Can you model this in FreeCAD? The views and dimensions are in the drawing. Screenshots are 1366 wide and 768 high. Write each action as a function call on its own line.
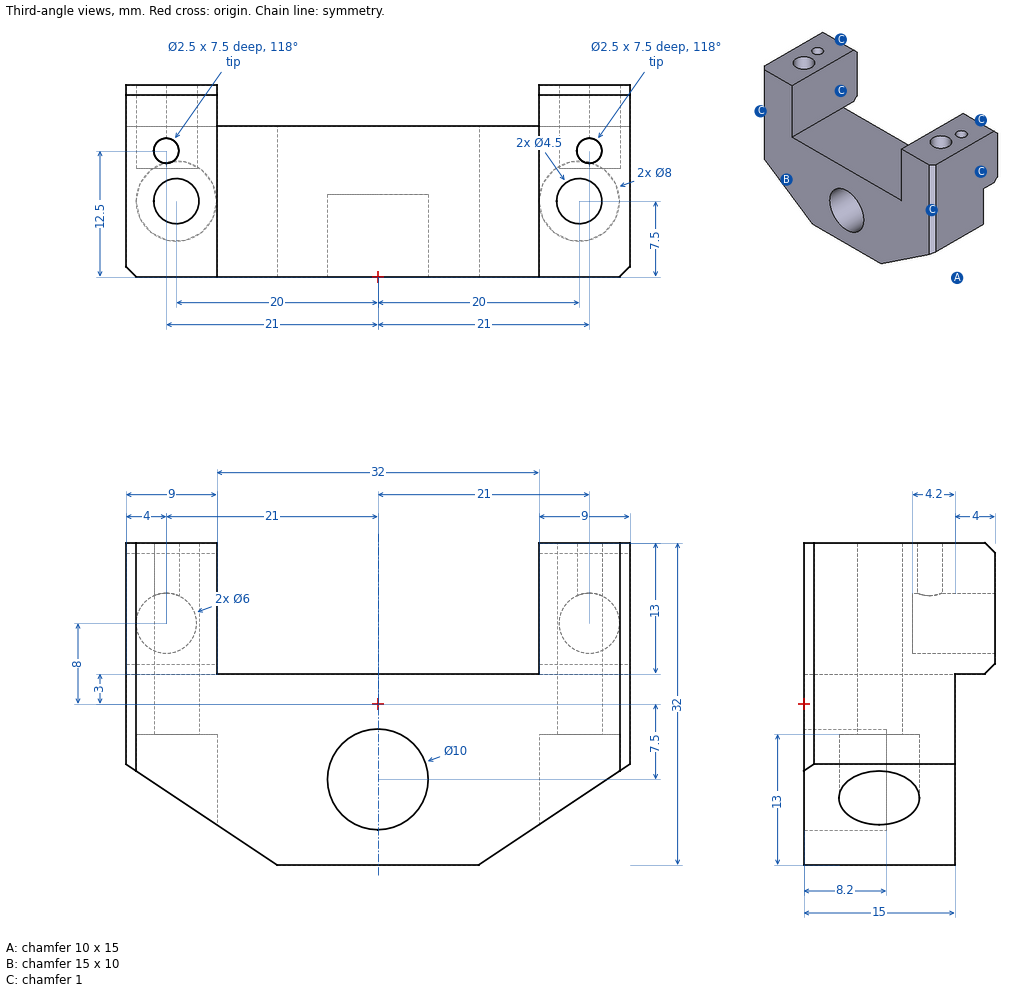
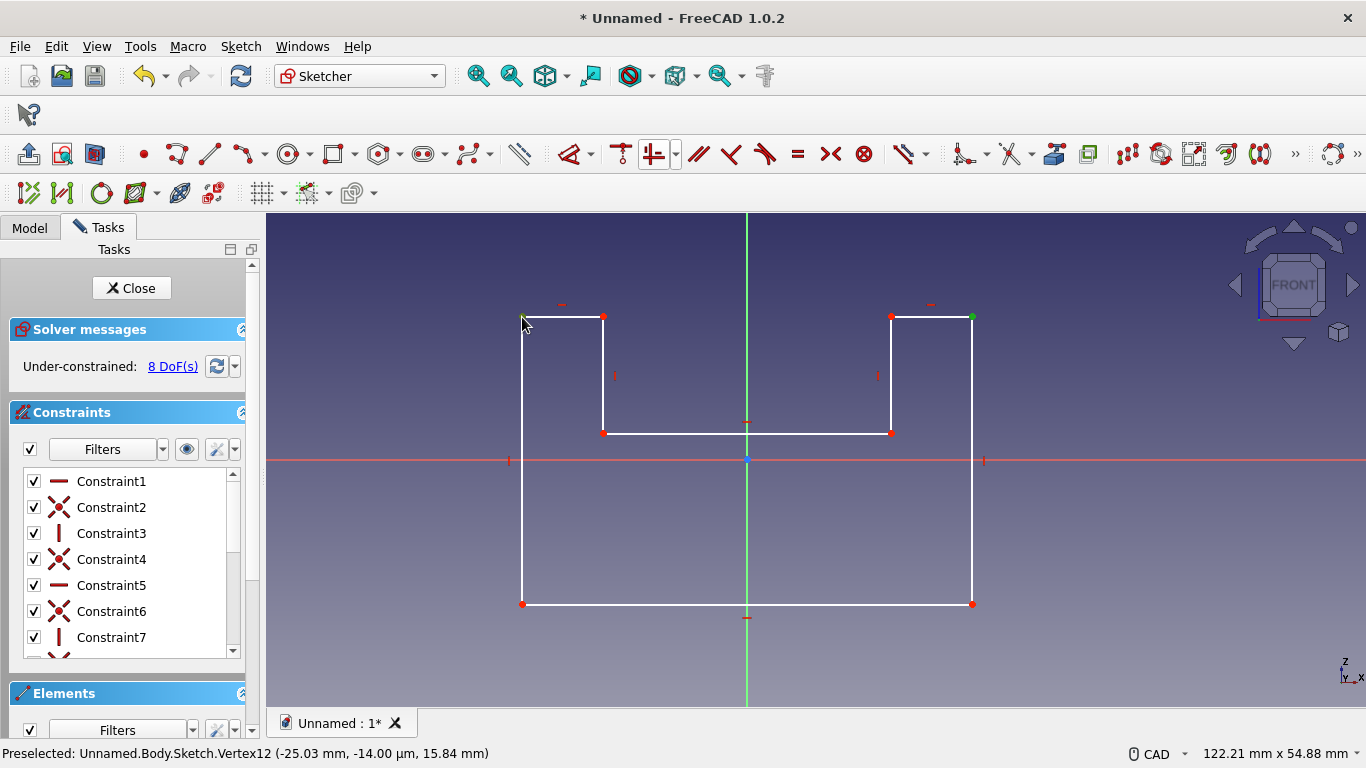
click(747, 648)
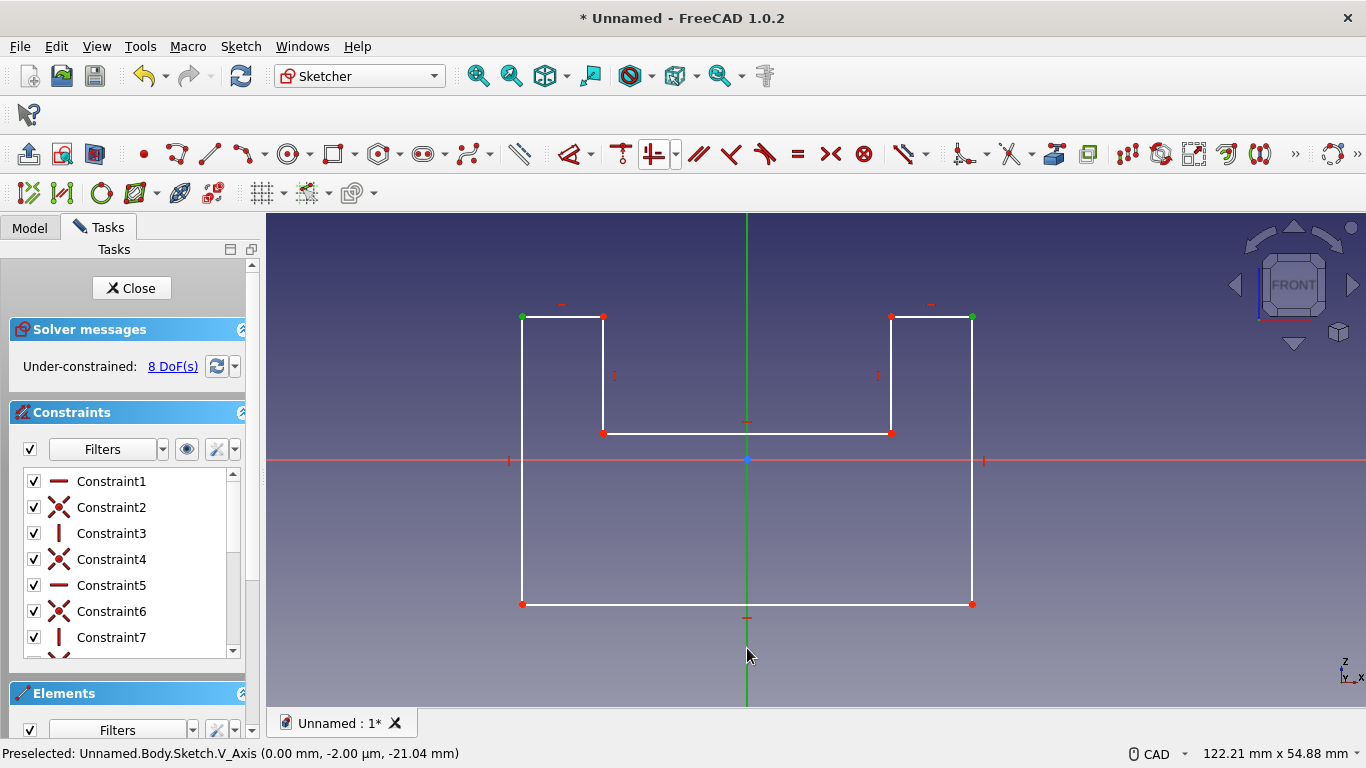
click(831, 154)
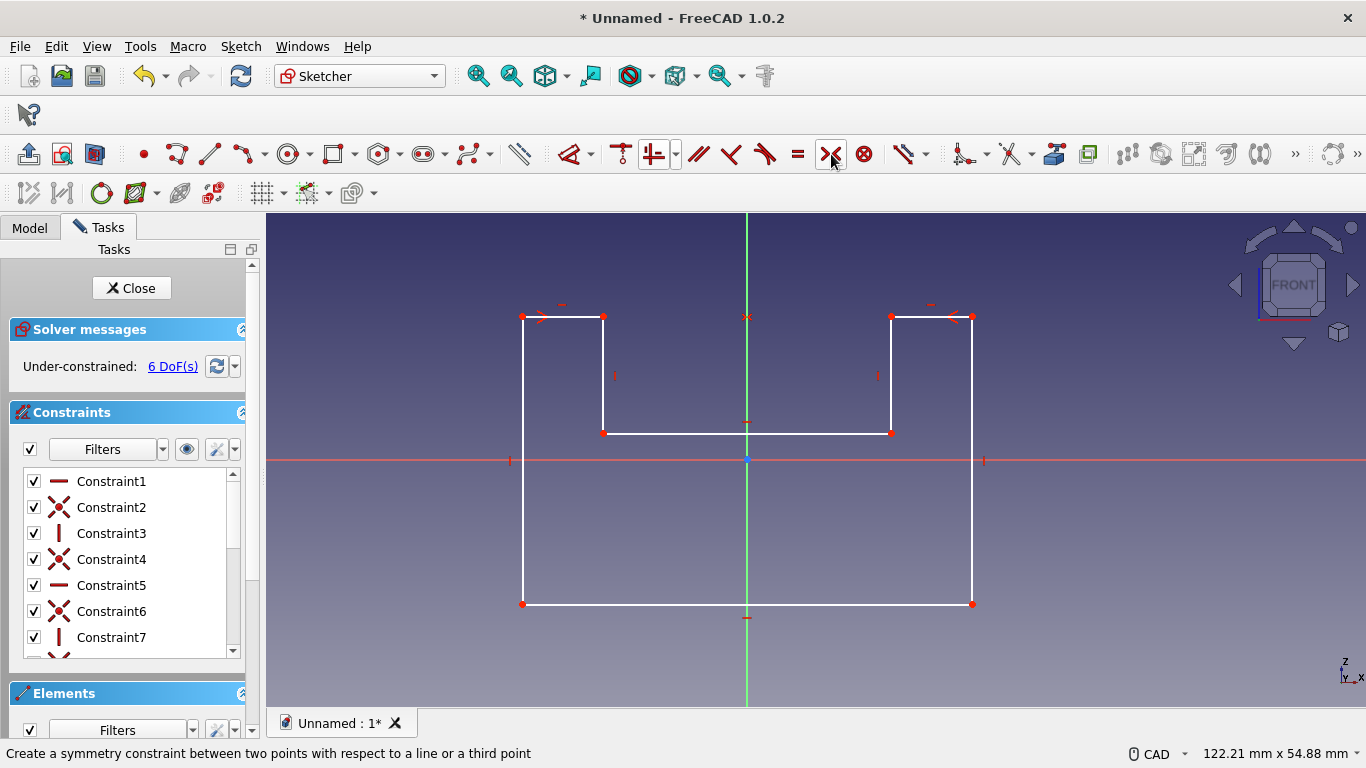
click(568, 154)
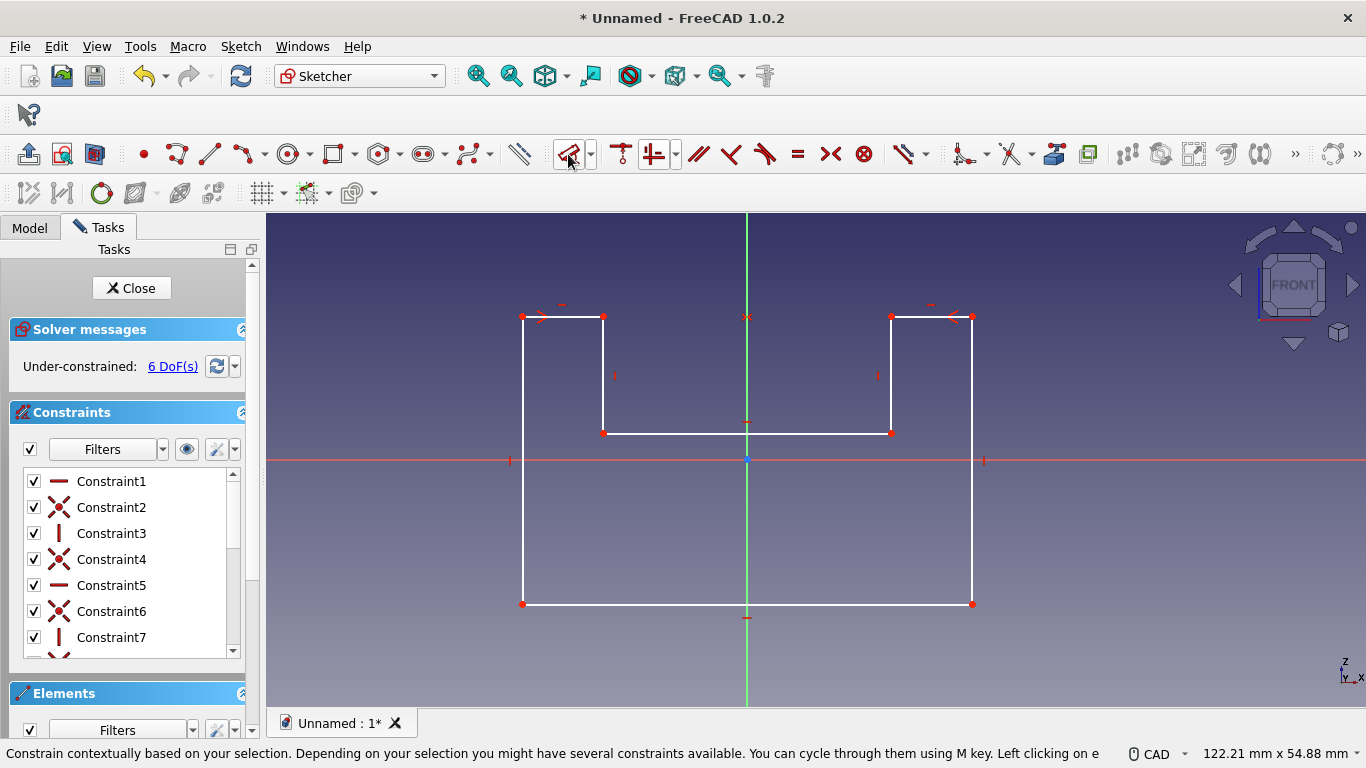
click(915, 317)
click(931, 283)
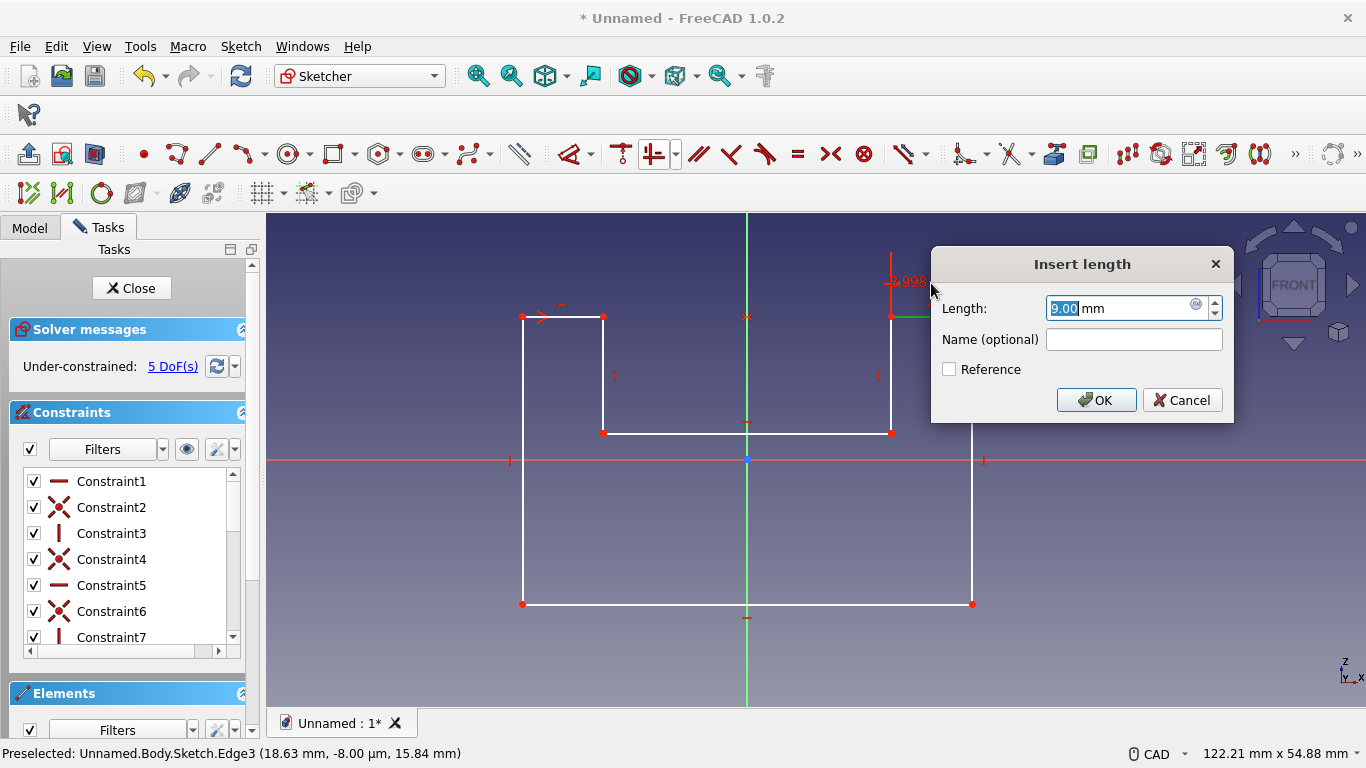
text(9)
key(Return)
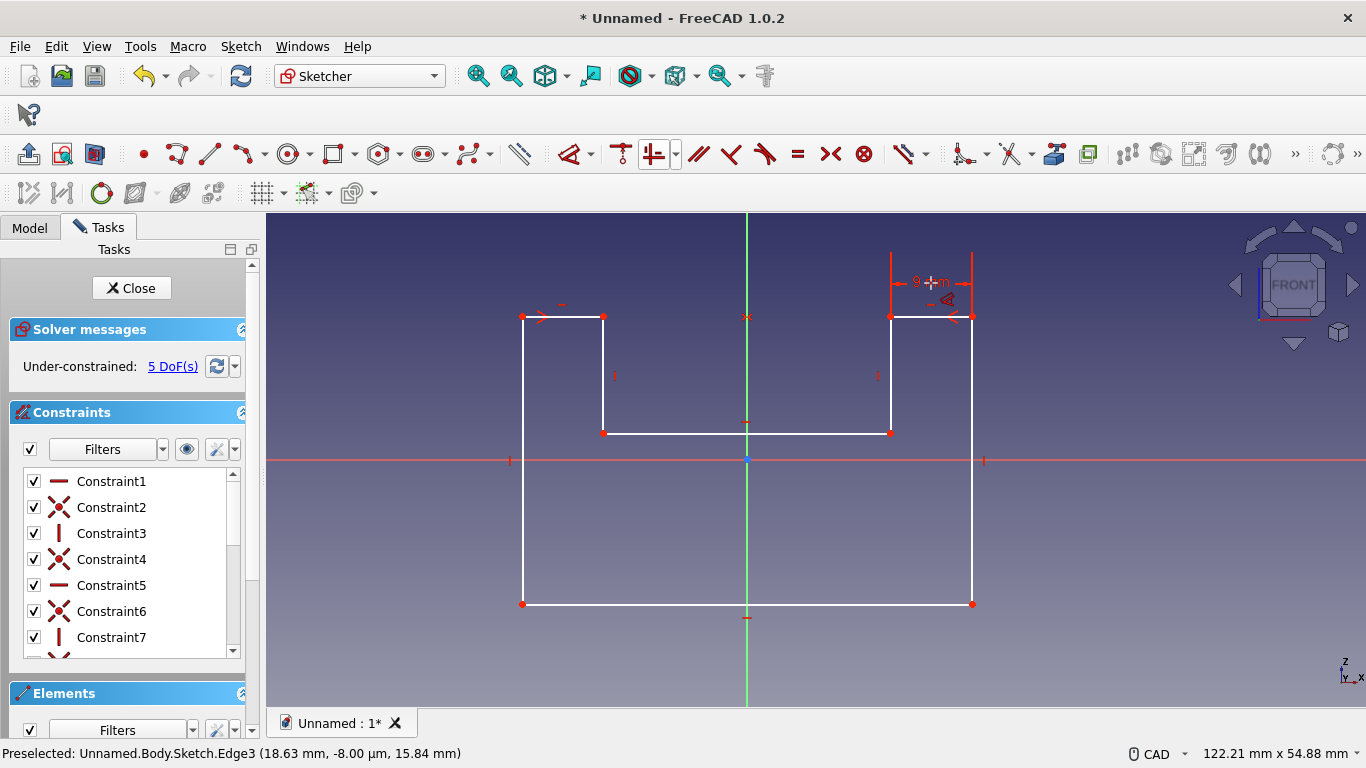
click(547, 317)
click(563, 283)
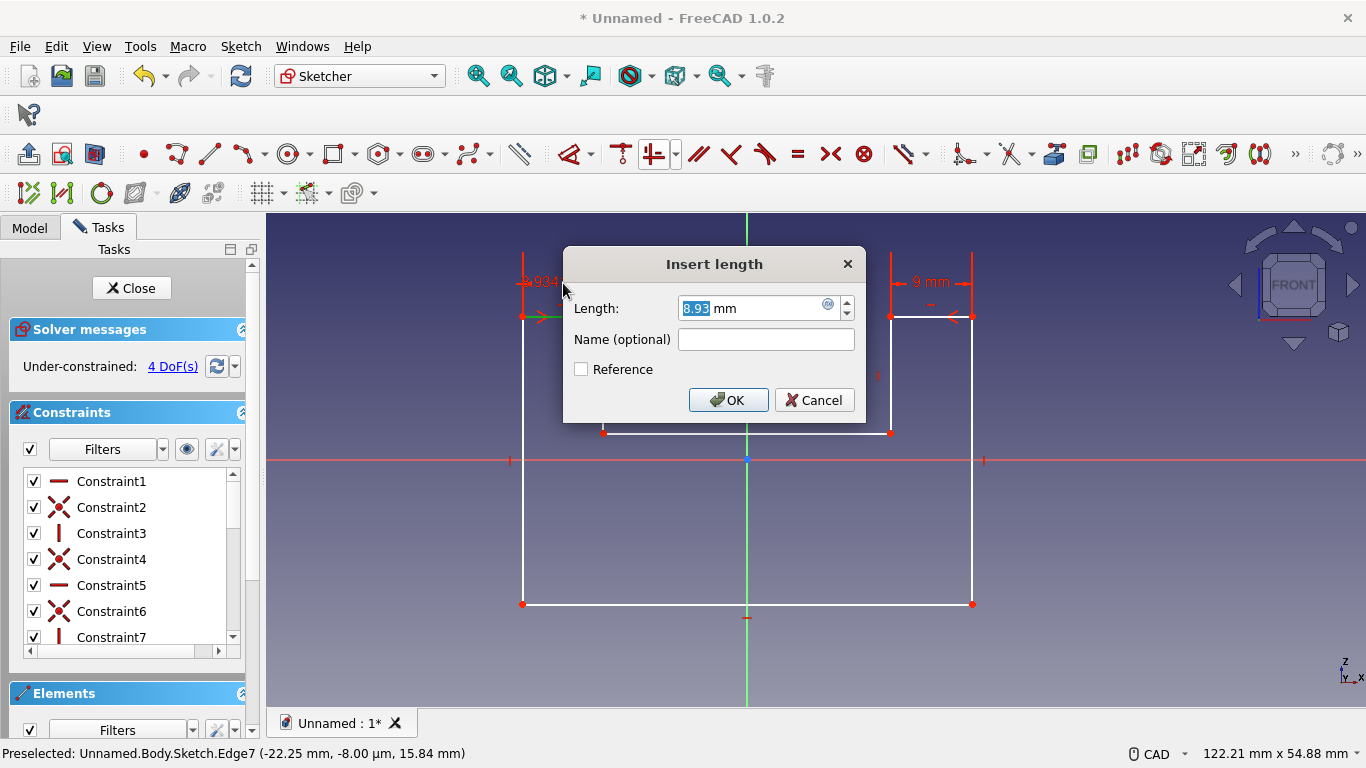
text(9)
key(Return)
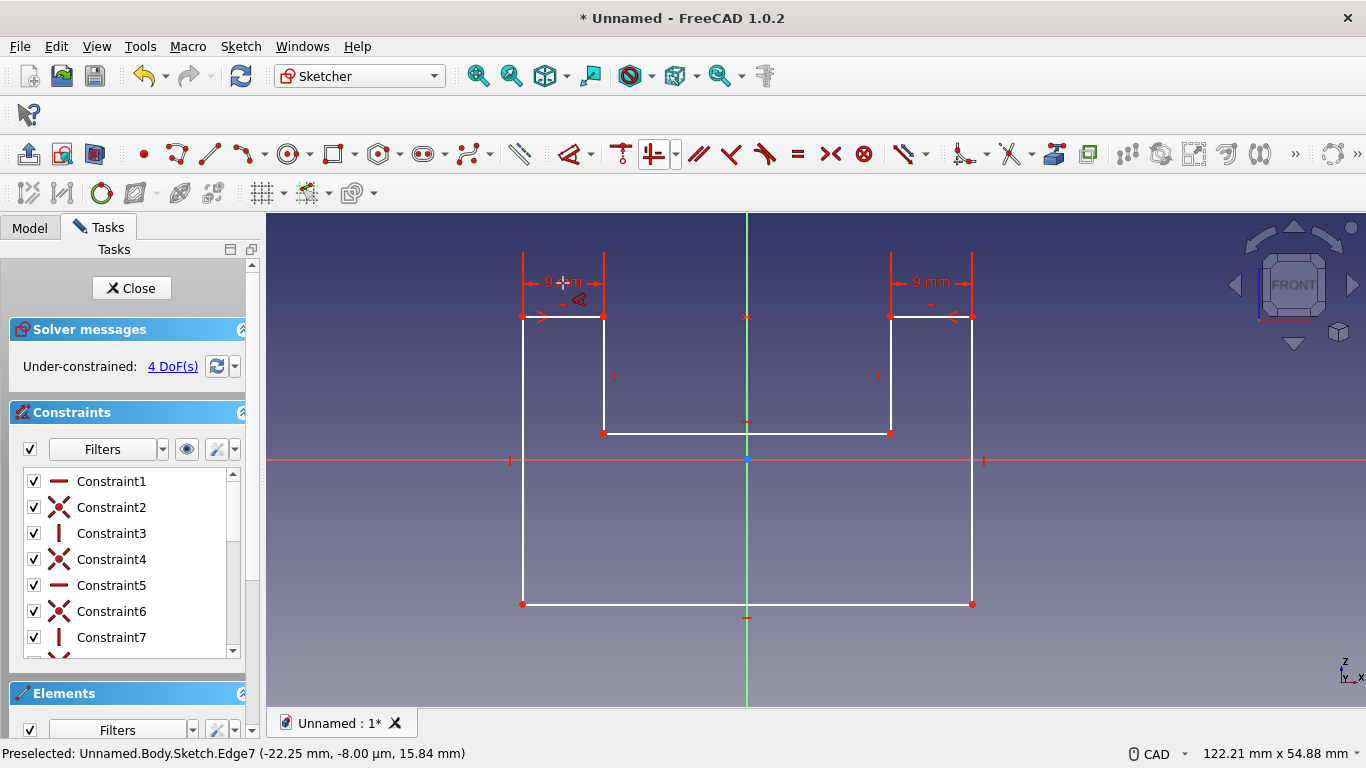
click(690, 434)
click(681, 400)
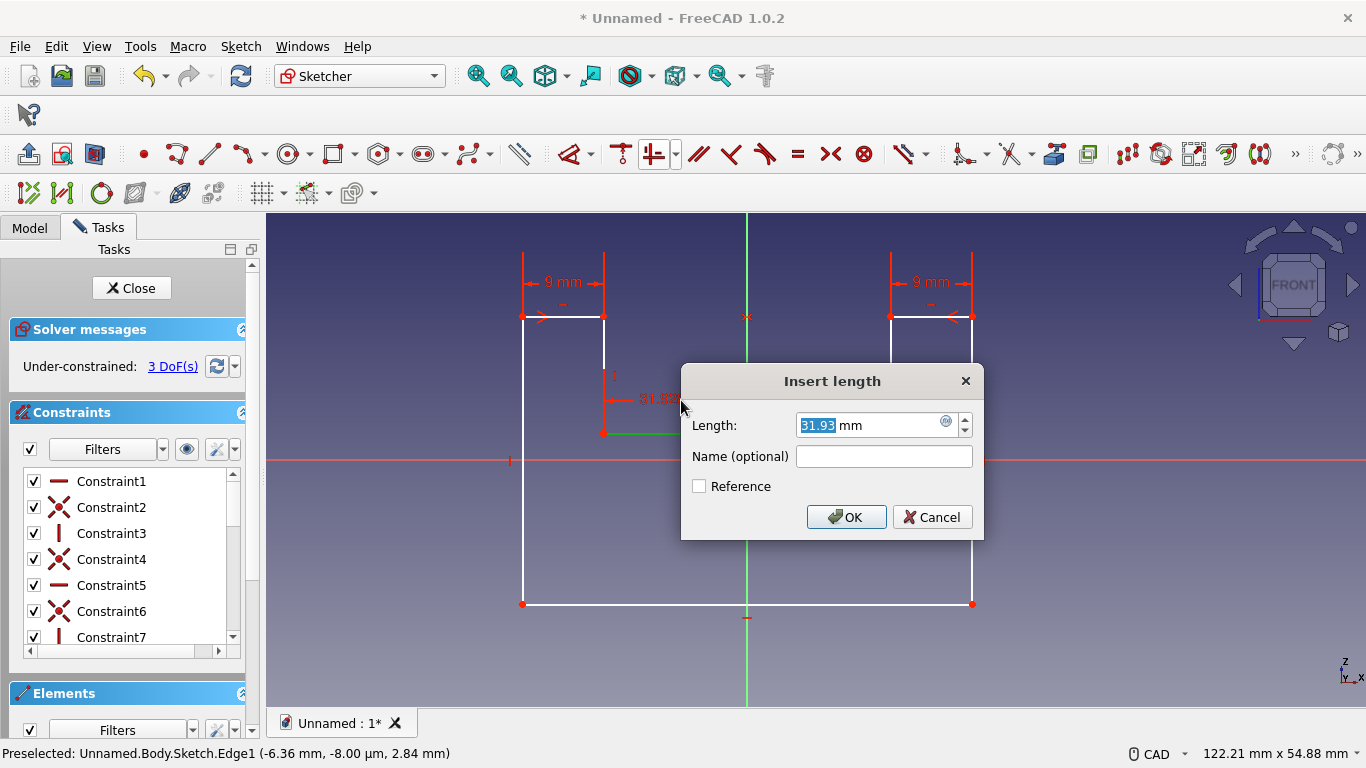
text(32)
key(Return)